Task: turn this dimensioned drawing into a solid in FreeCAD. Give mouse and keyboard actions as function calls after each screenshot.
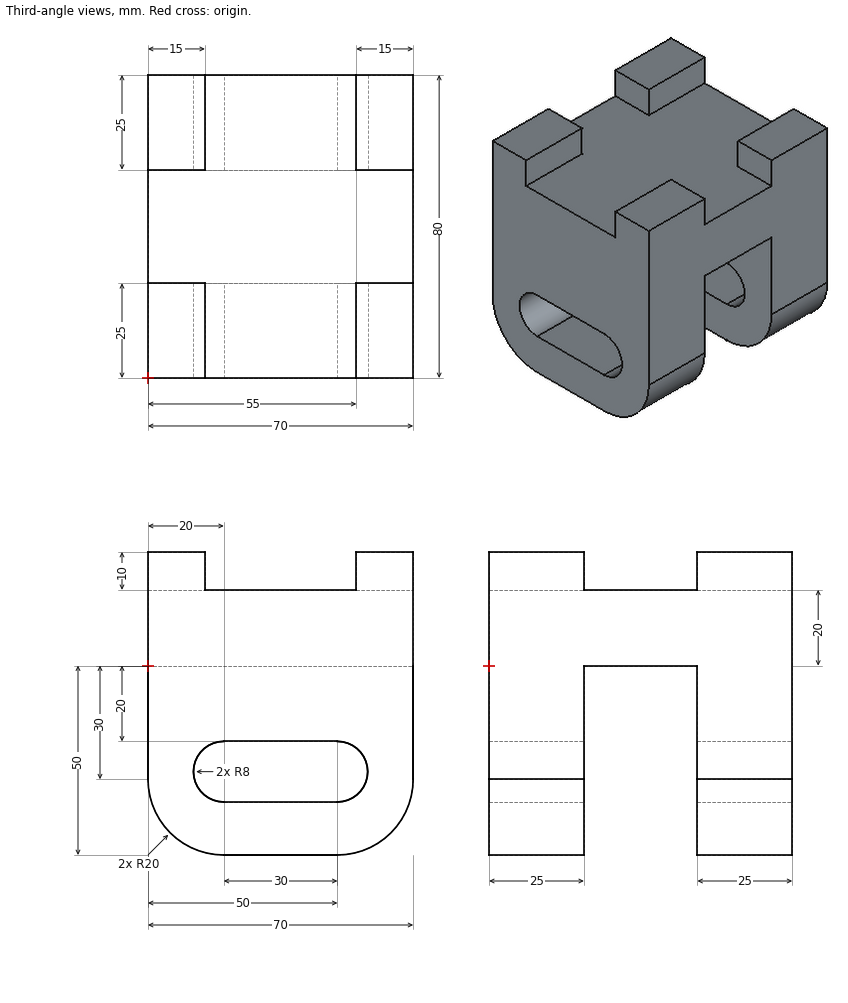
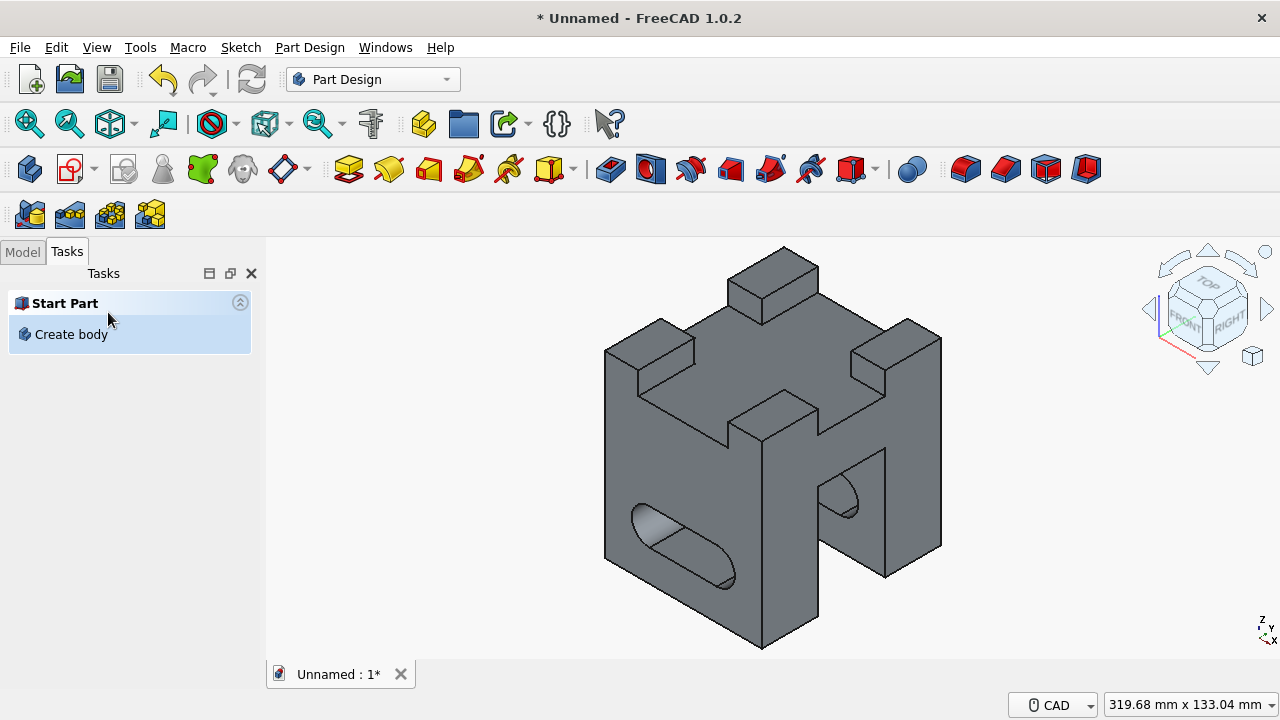
click(706, 482)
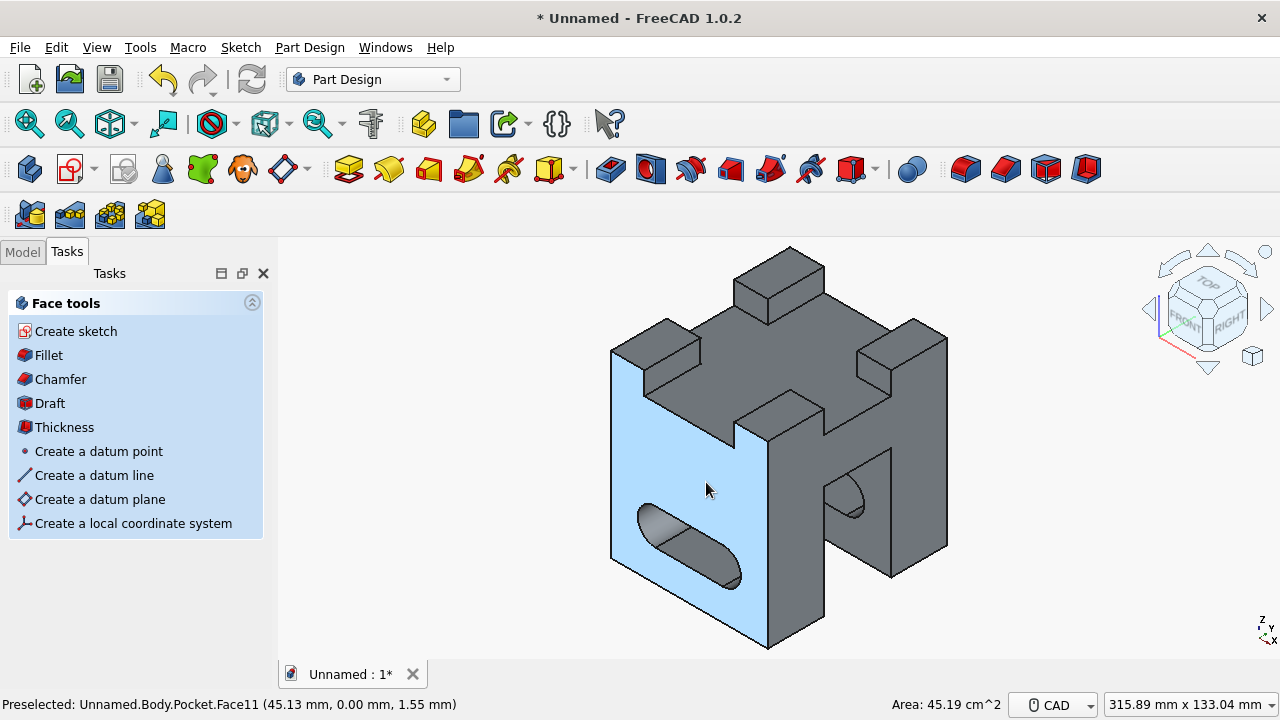
click(70, 170)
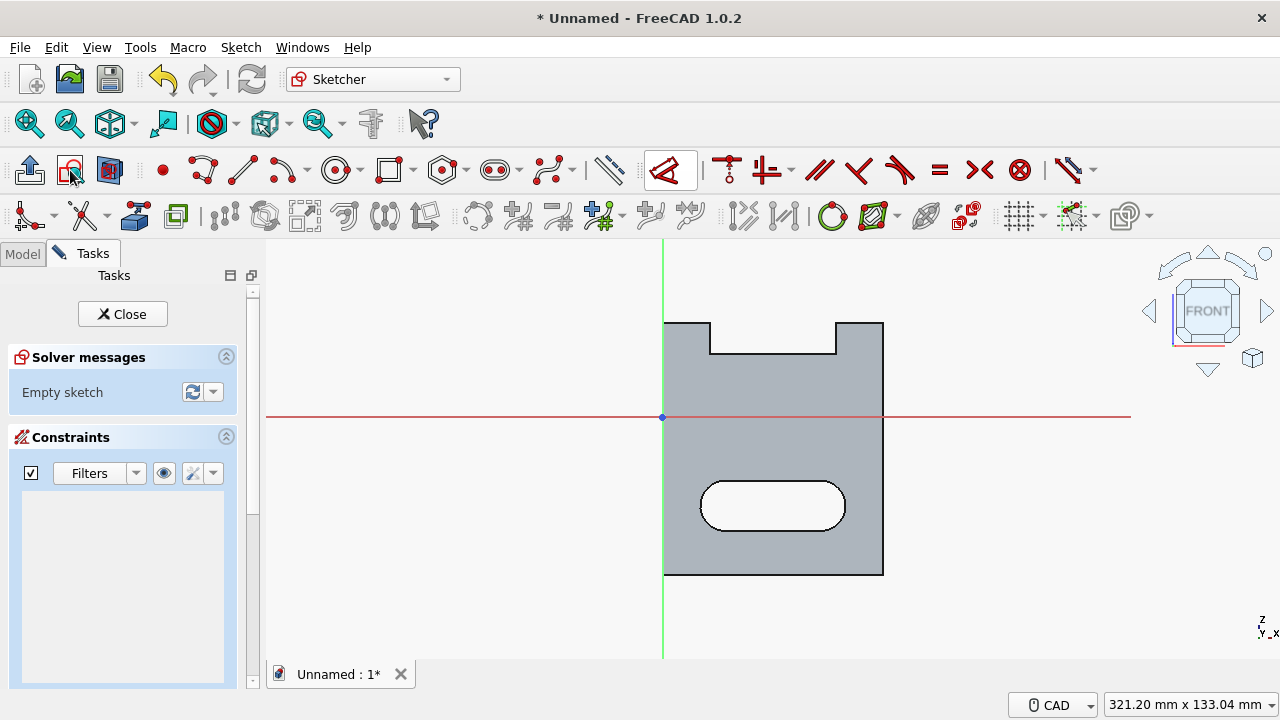
scroll(912, 593, up, 2)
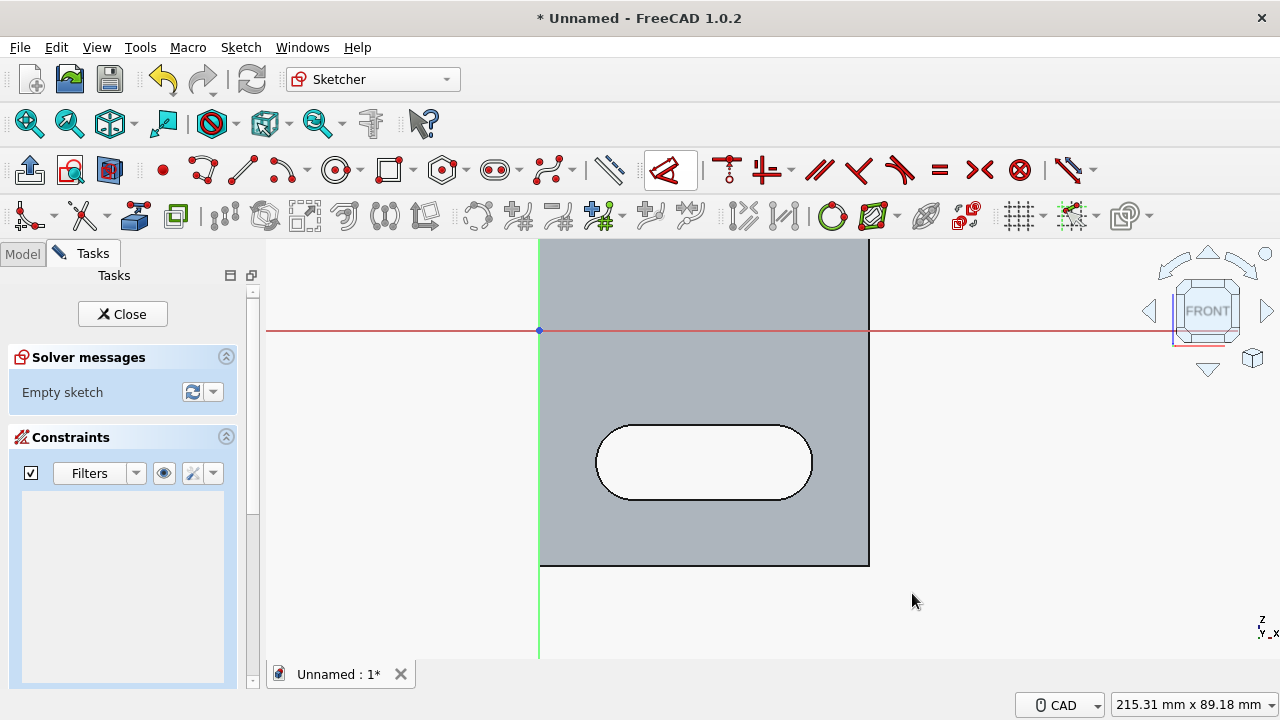
click(204, 170)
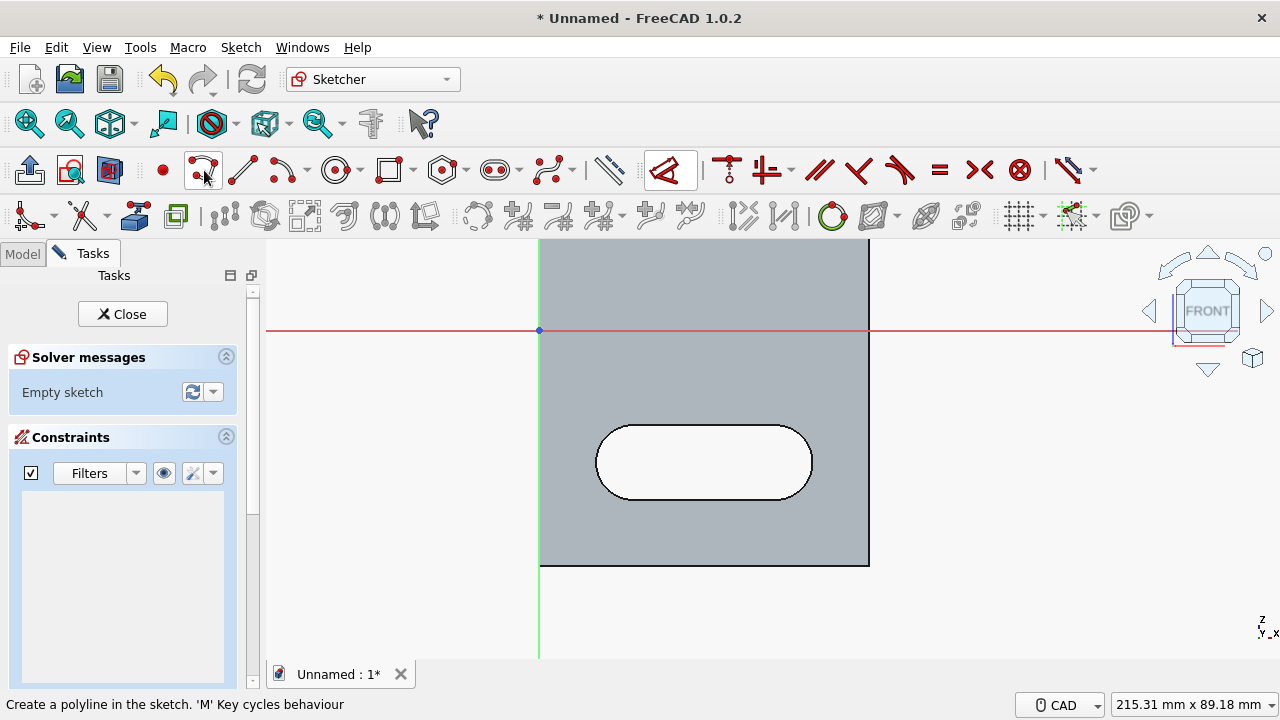
click(539, 472)
click(548, 566)
click(634, 566)
right_click(634, 566)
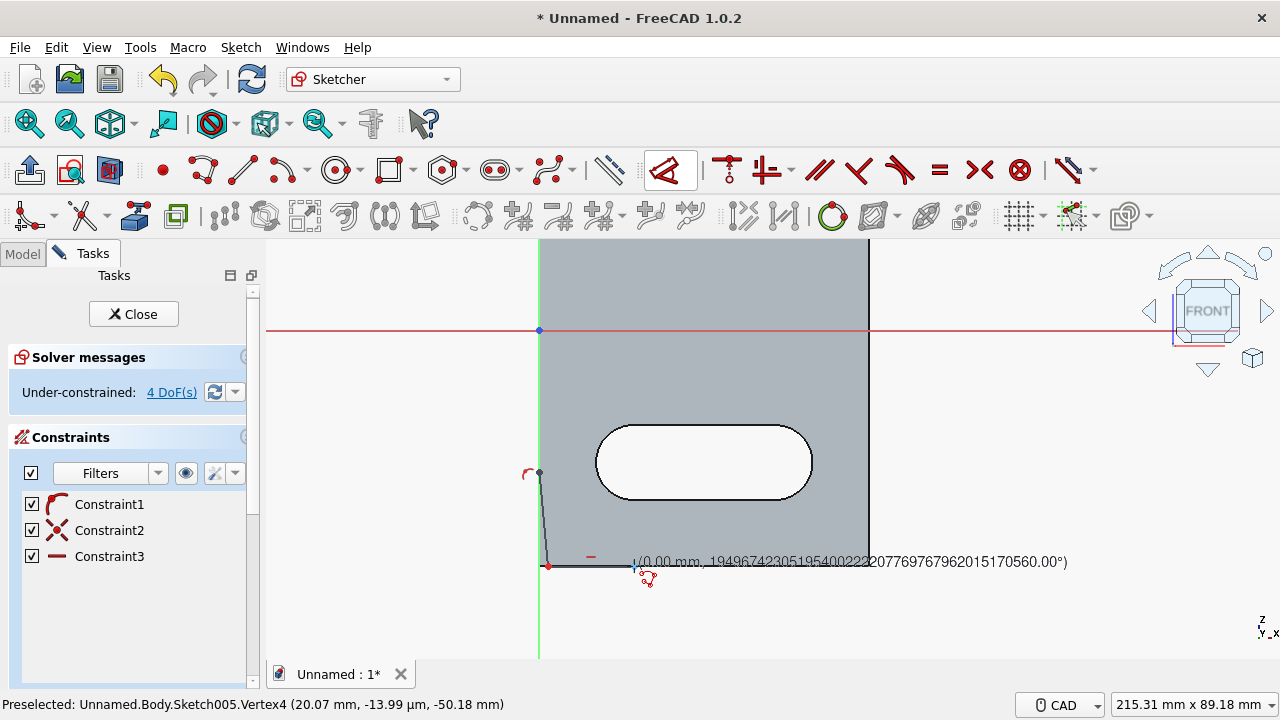
click(310, 170)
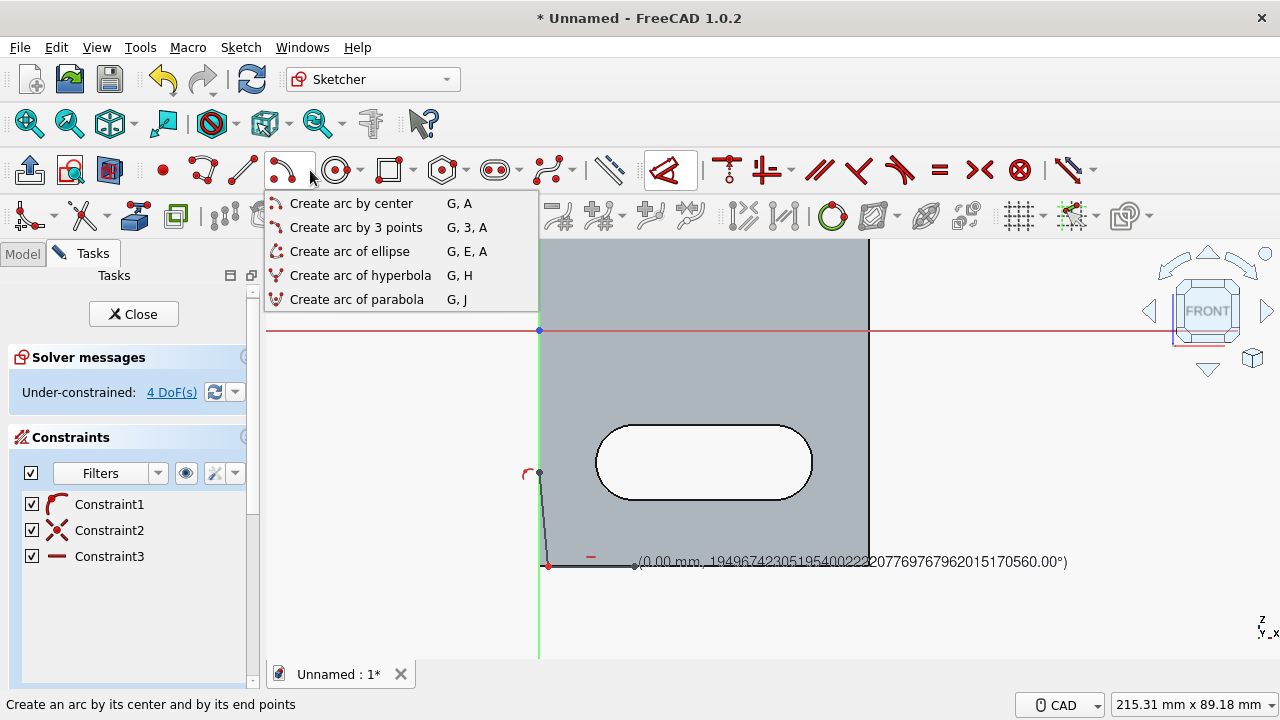
click(402, 227)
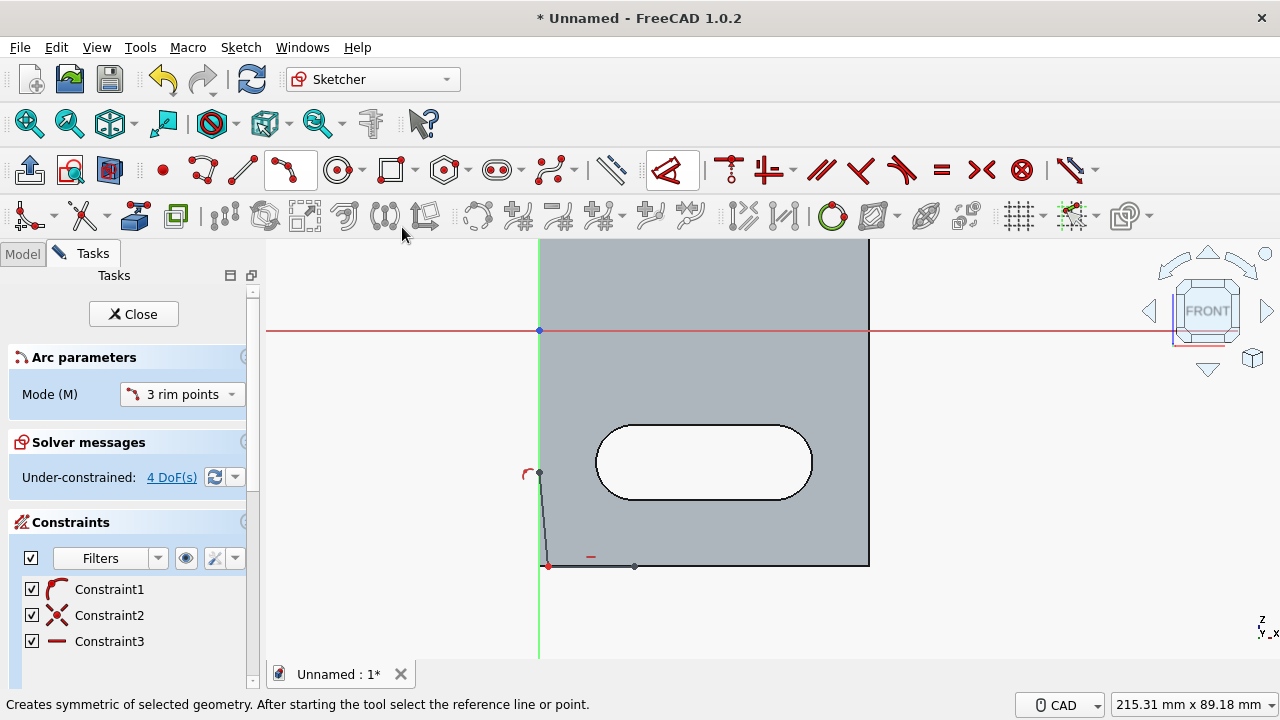
click(634, 567)
click(539, 473)
click(567, 539)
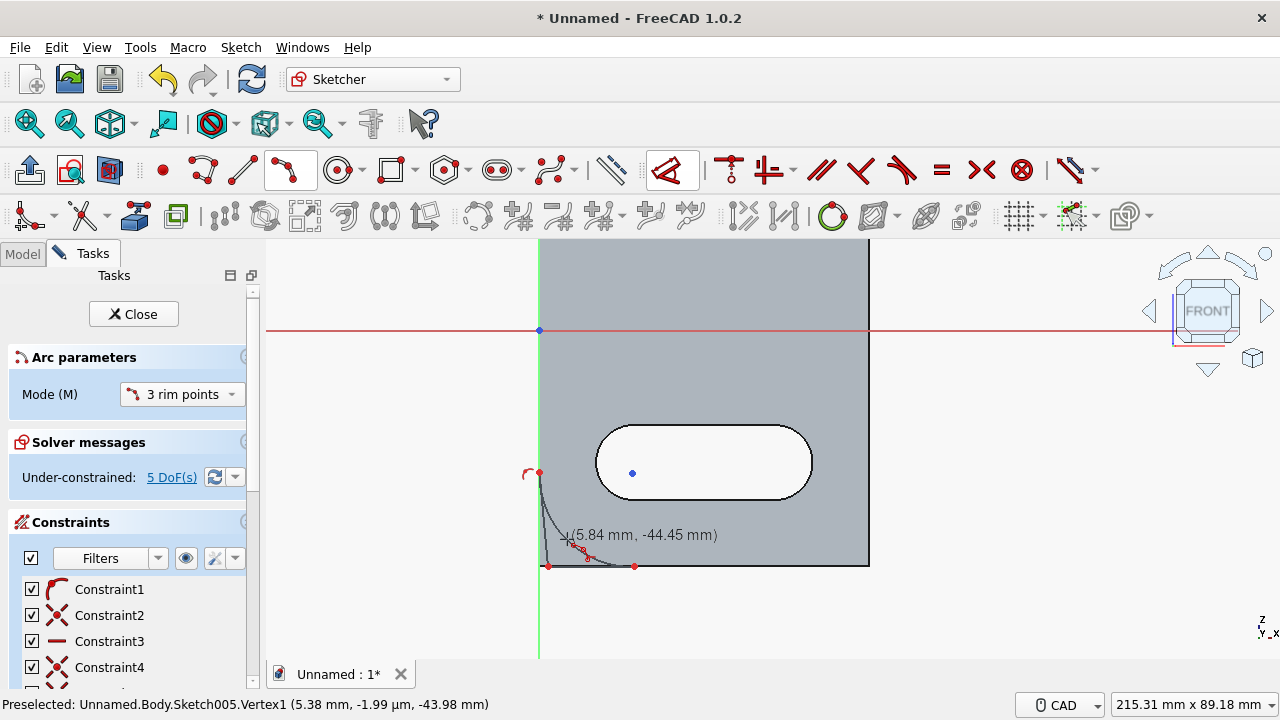
click(204, 170)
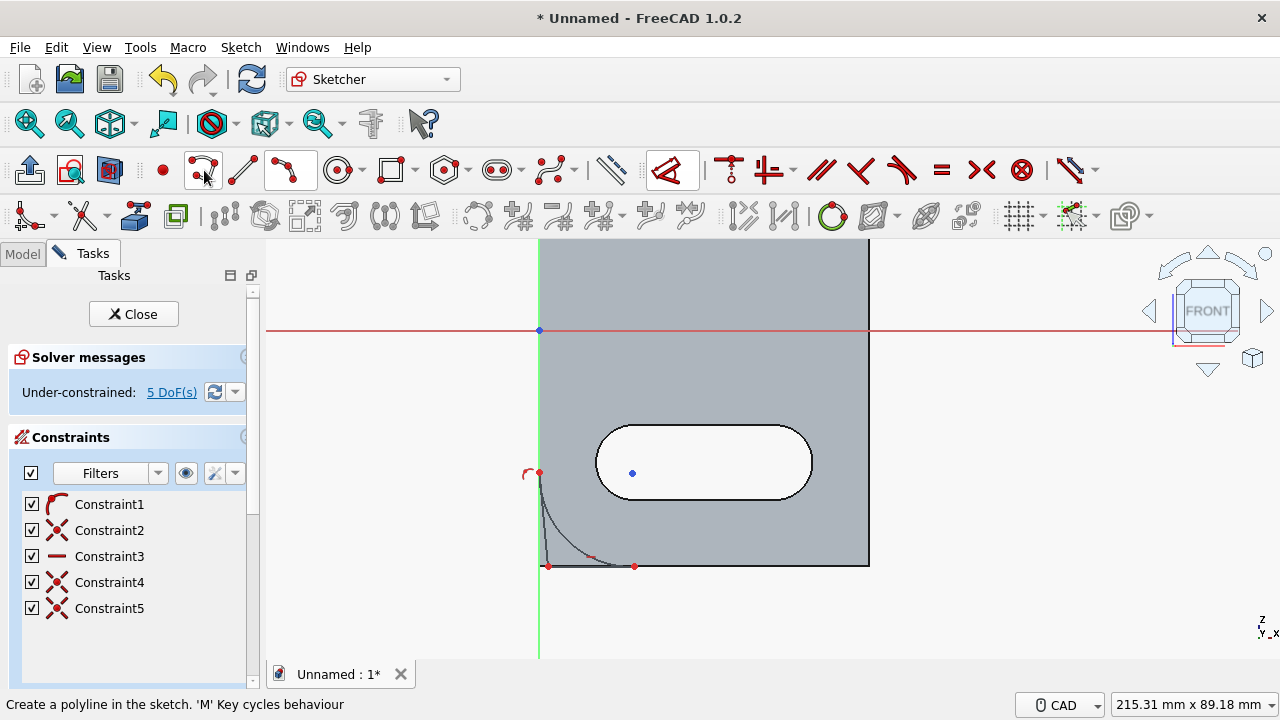
click(775, 566)
click(869, 566)
click(869, 472)
right_click(869, 472)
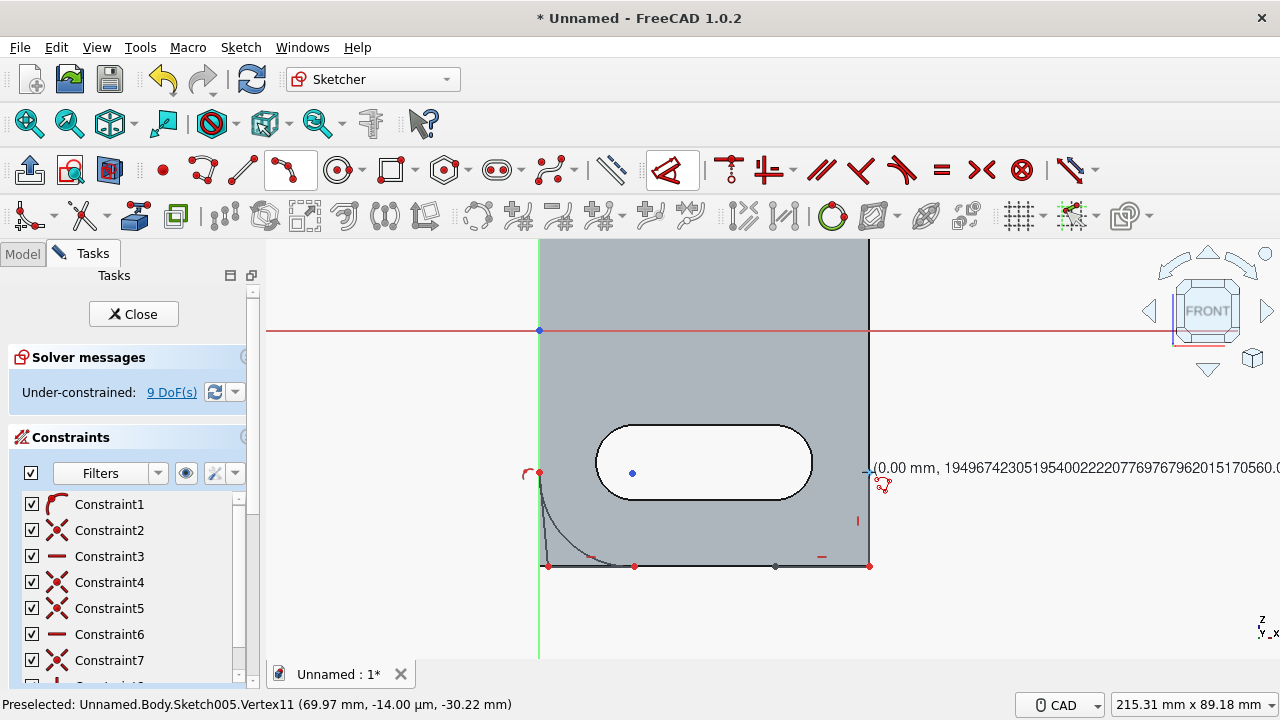
click(284, 170)